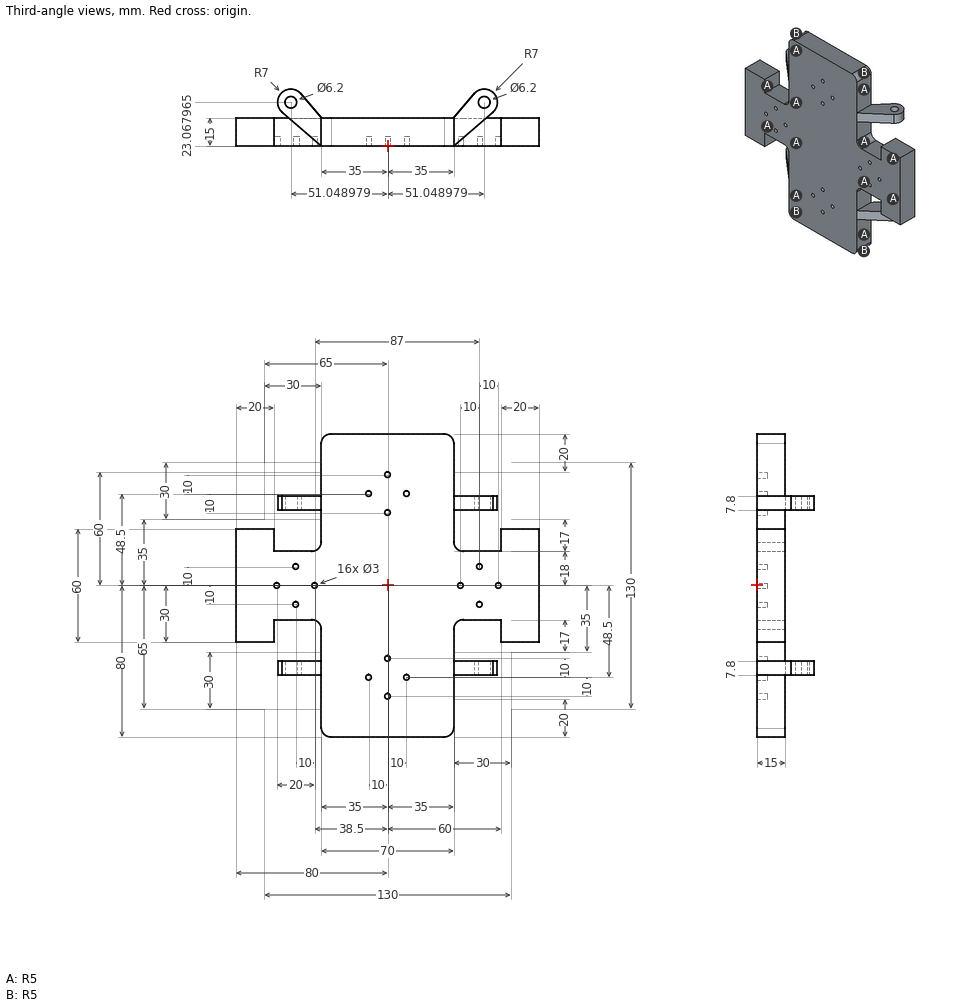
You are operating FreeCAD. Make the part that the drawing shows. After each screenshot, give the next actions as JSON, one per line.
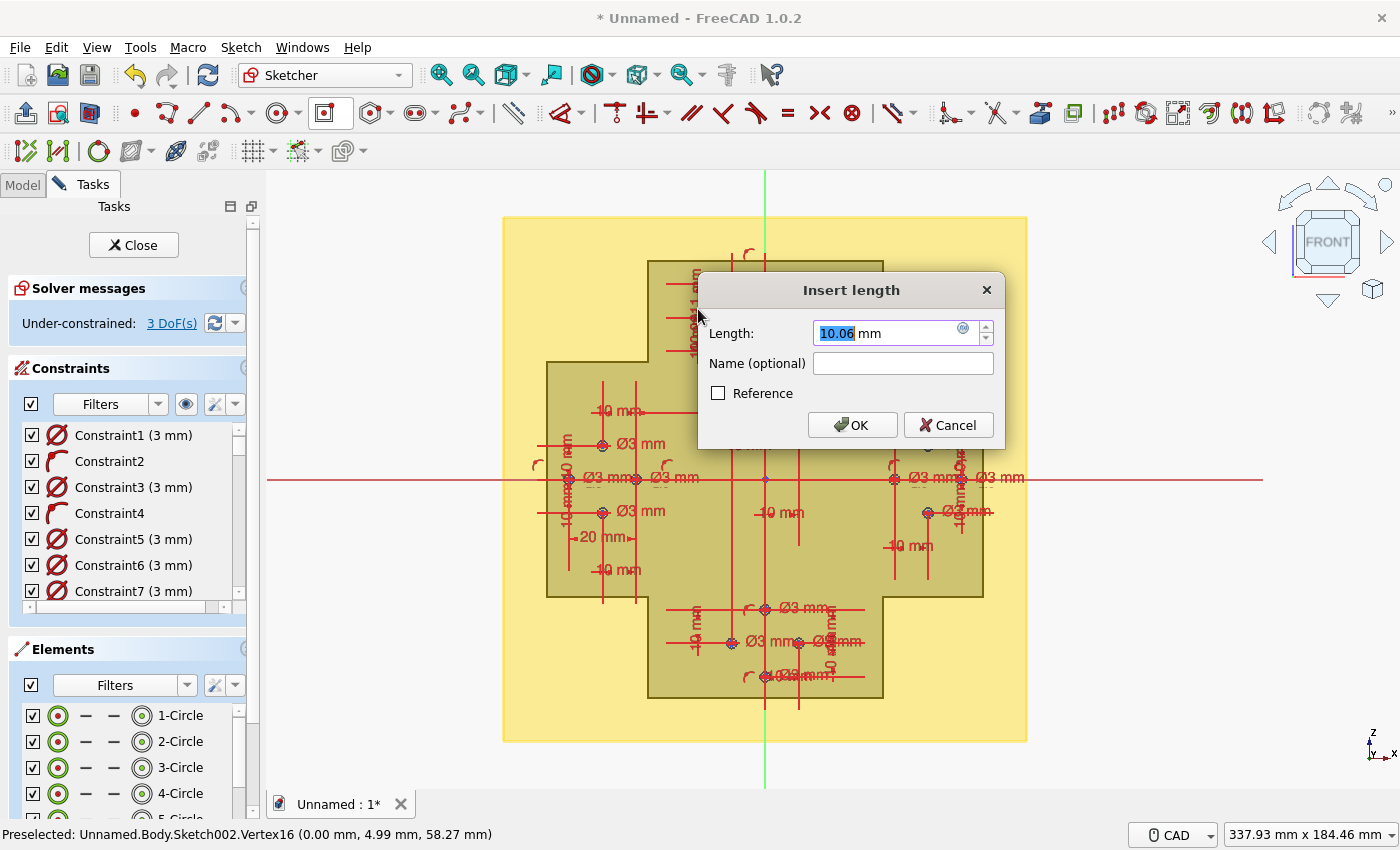
{"action": "type", "text": "10"}
{"action": "key", "text": "Return"}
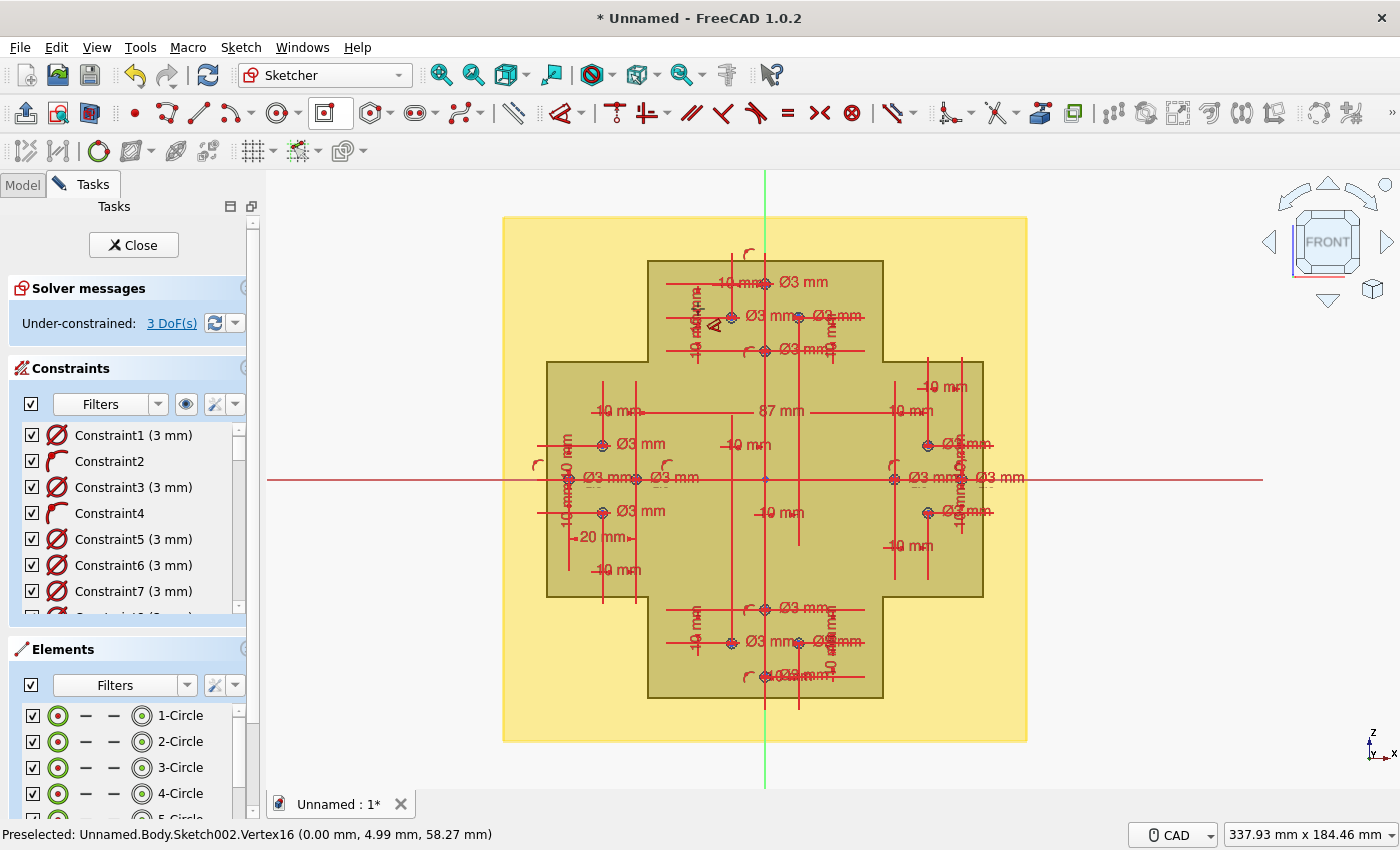
{"action": "left_click", "coordinate": [636, 480]}
{"action": "left_click", "coordinate": [701, 514]}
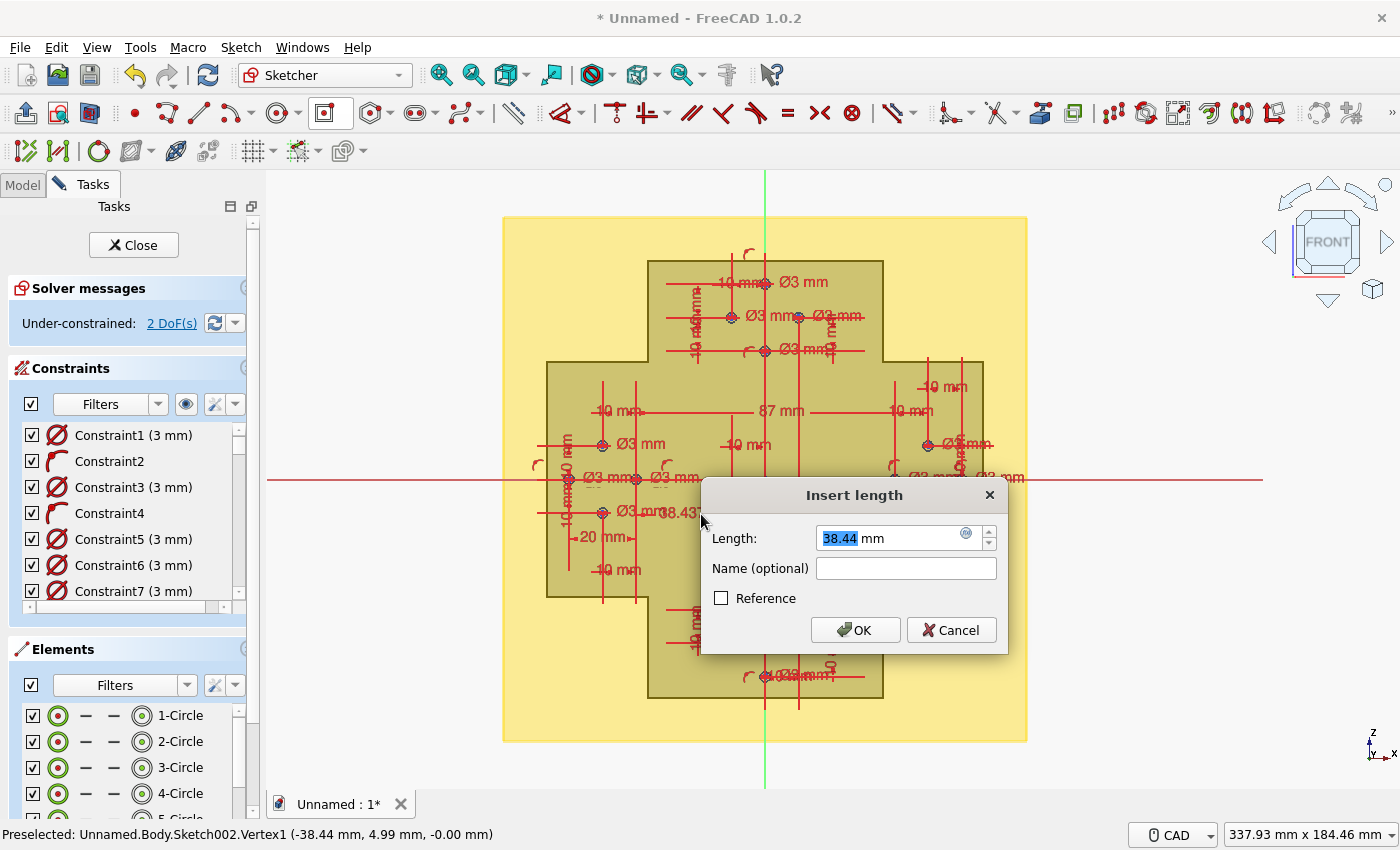
{"action": "type", "text": "38.5"}
{"action": "key", "text": "Return"}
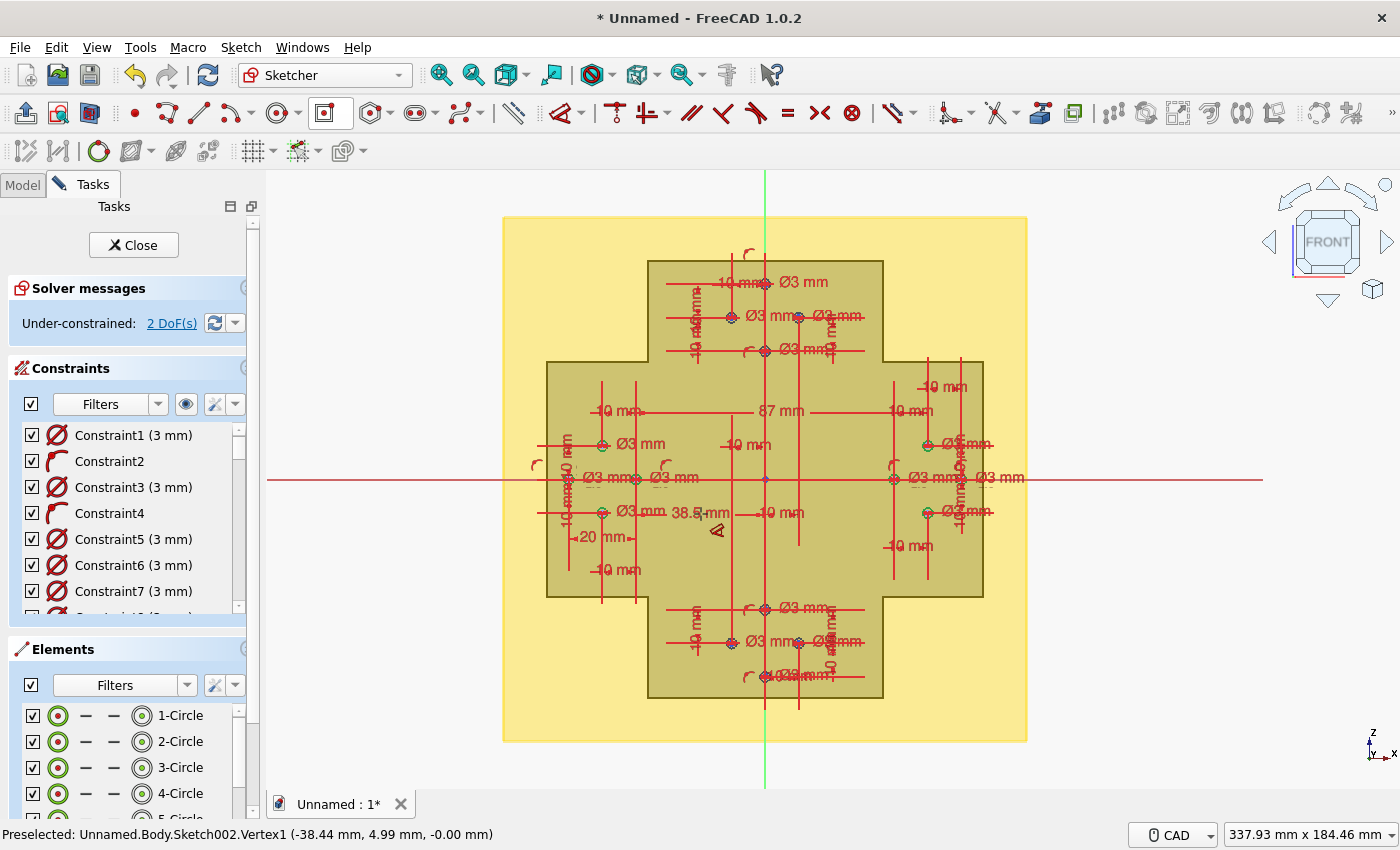
{"action": "left_click", "coordinate": [799, 643]}
{"action": "left_click", "coordinate": [833, 561]}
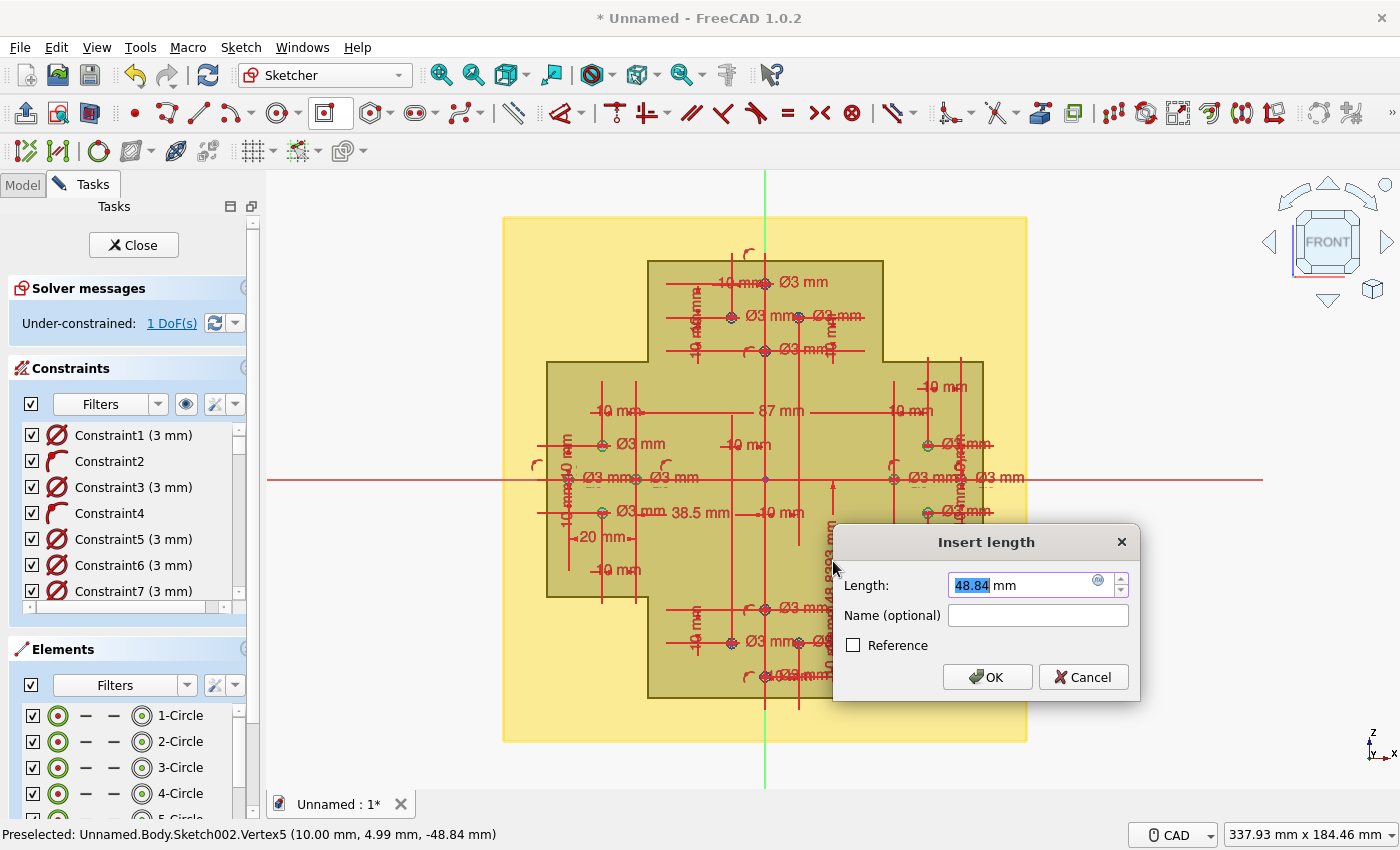
{"action": "type", "text": "48.5"}
{"action": "key", "text": "Return"}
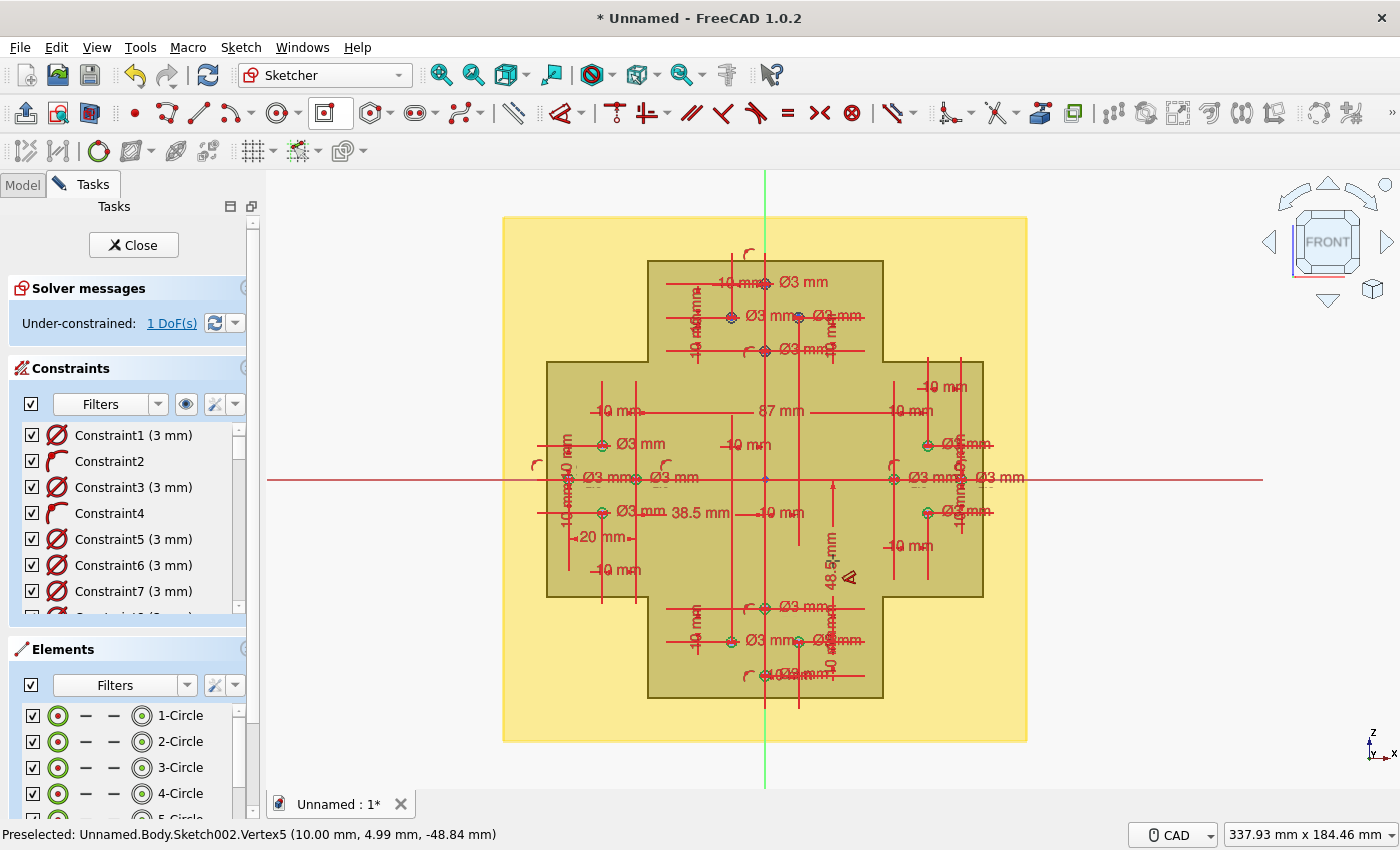
{"action": "left_click", "coordinate": [732, 318]}
{"action": "left_click", "coordinate": [698, 399]}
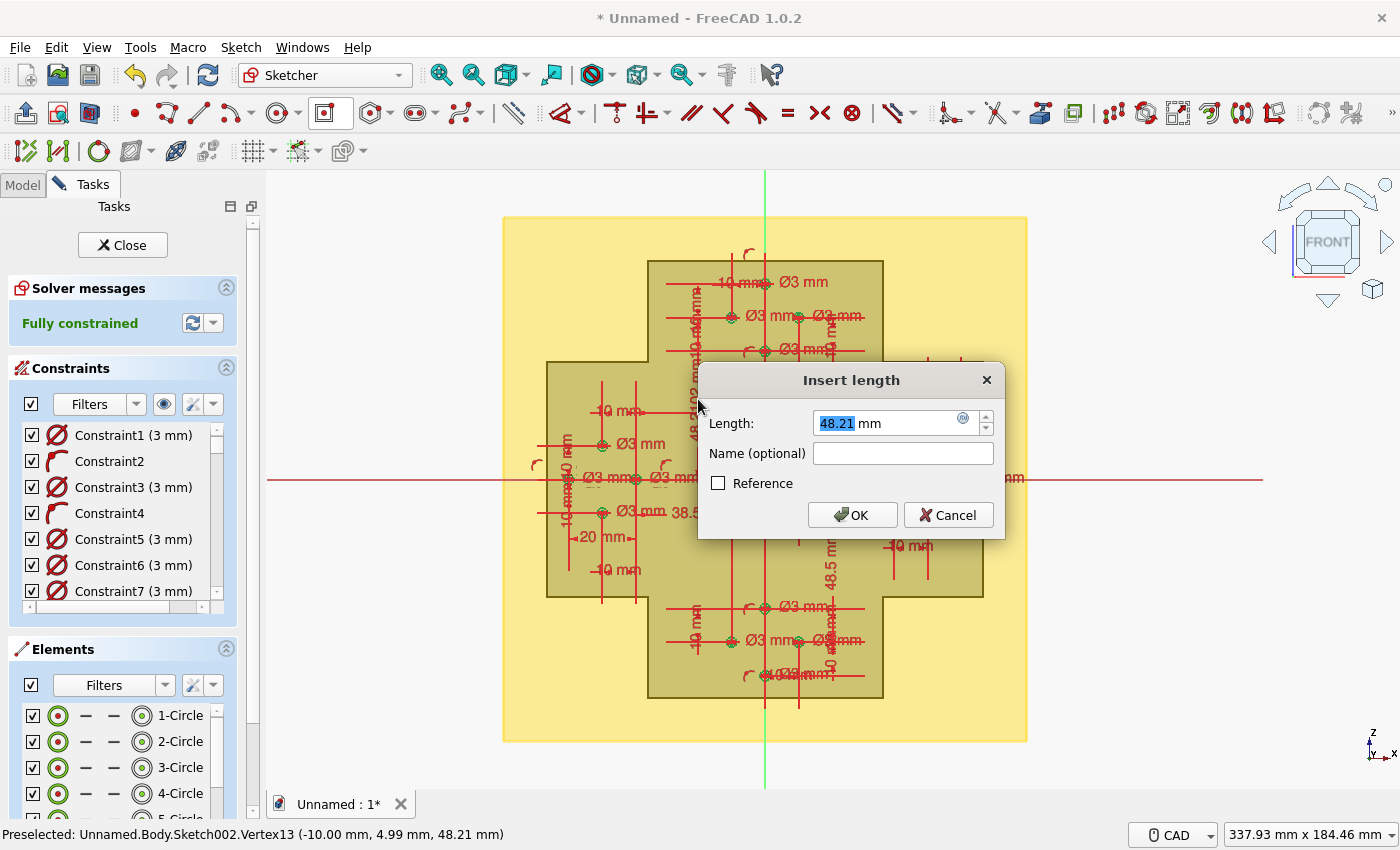
{"action": "type", "text": "48.5"}
{"action": "key", "text": "Return"}
{"action": "key", "text": "Escape"}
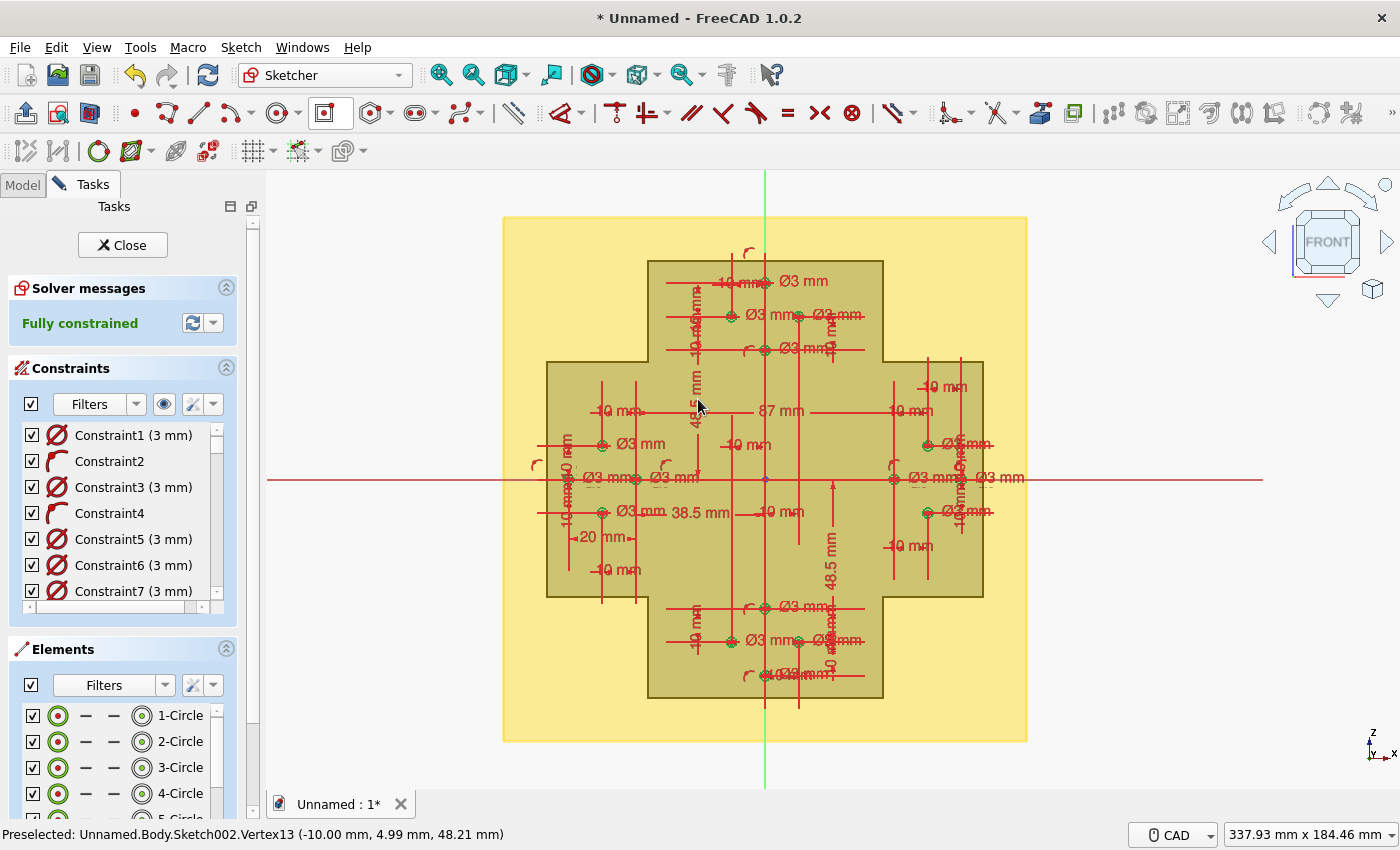
{"action": "left_click", "coordinate": [123, 245]}